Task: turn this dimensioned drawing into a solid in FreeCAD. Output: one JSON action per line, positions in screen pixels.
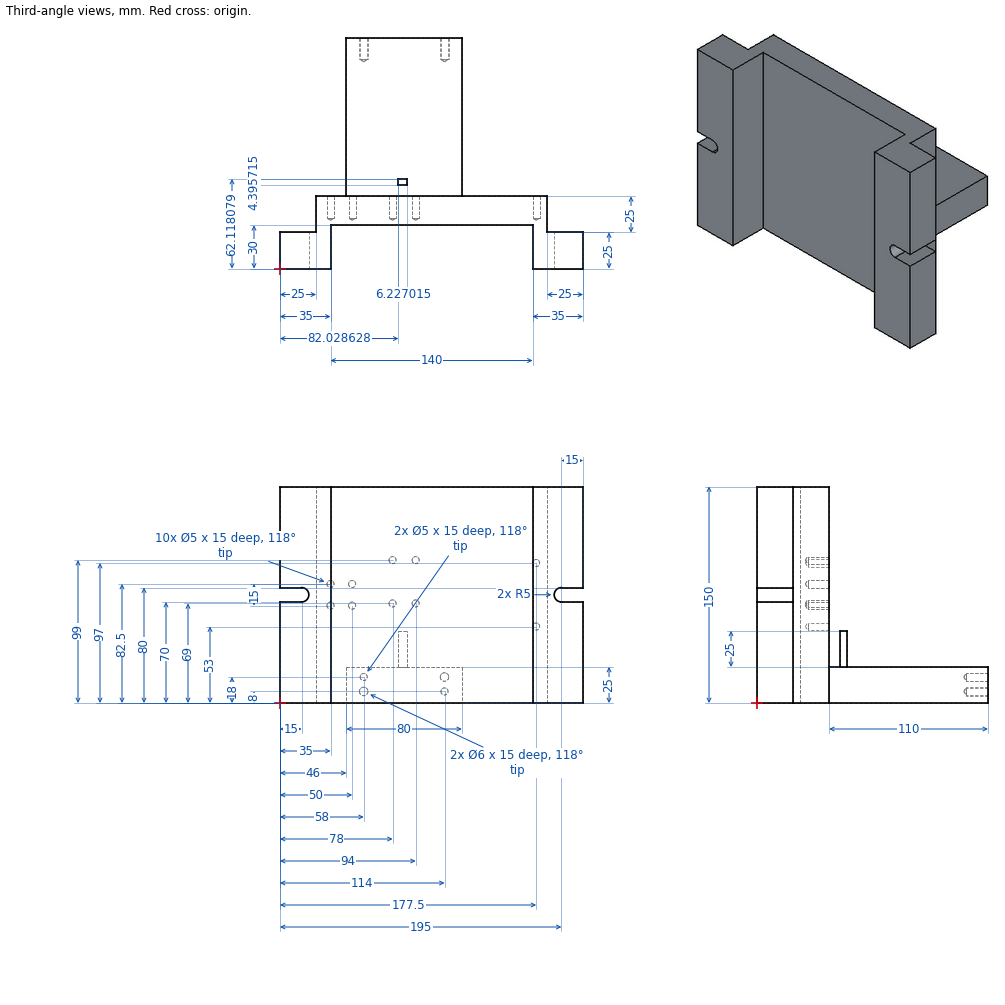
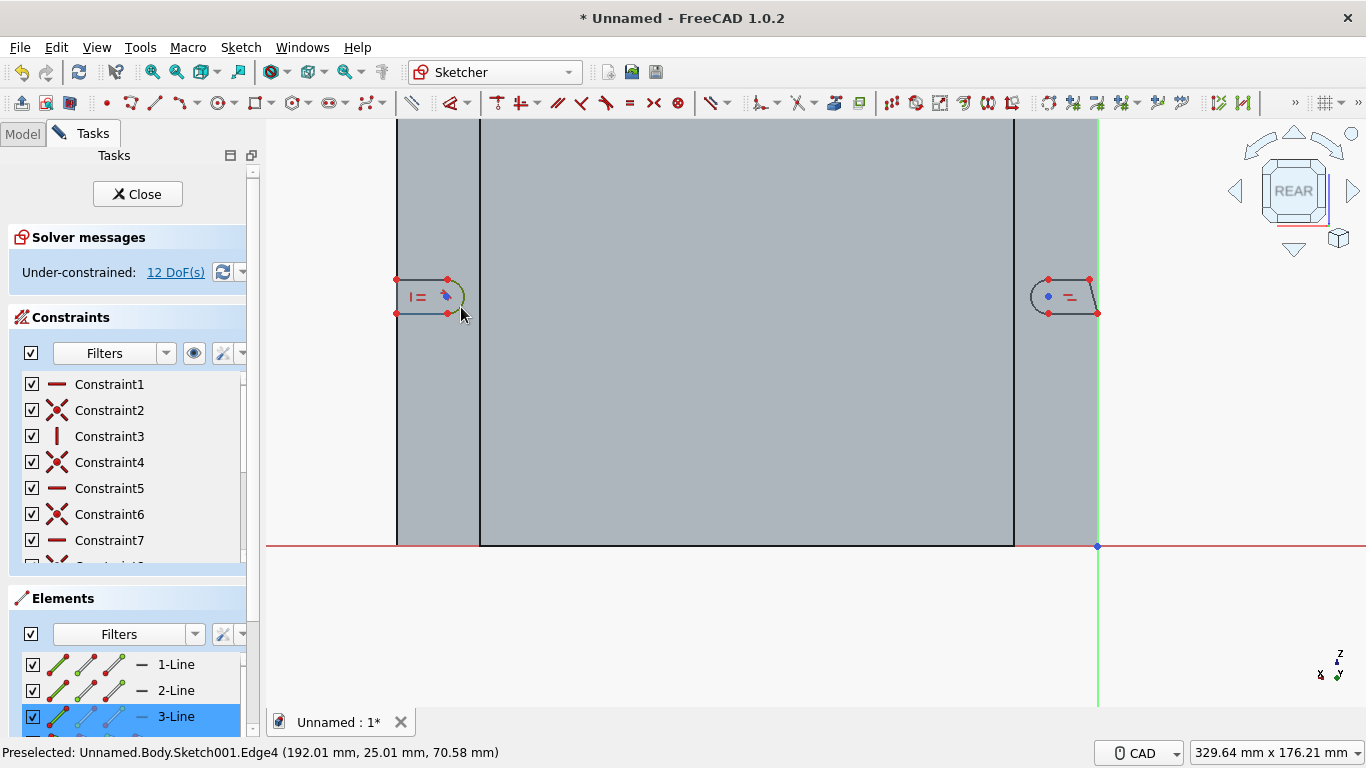
{"action": "key", "text": "t"}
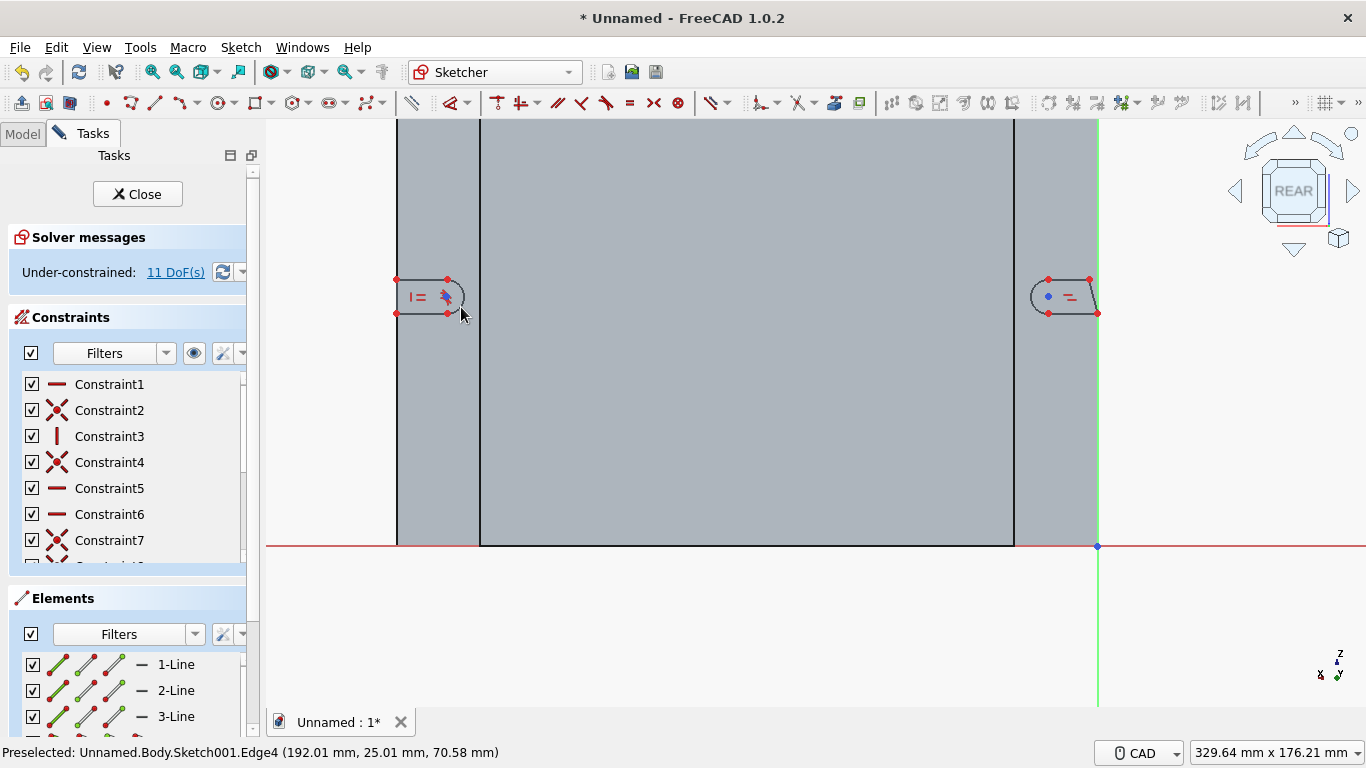
{"action": "left_click", "coordinate": [1063, 314]}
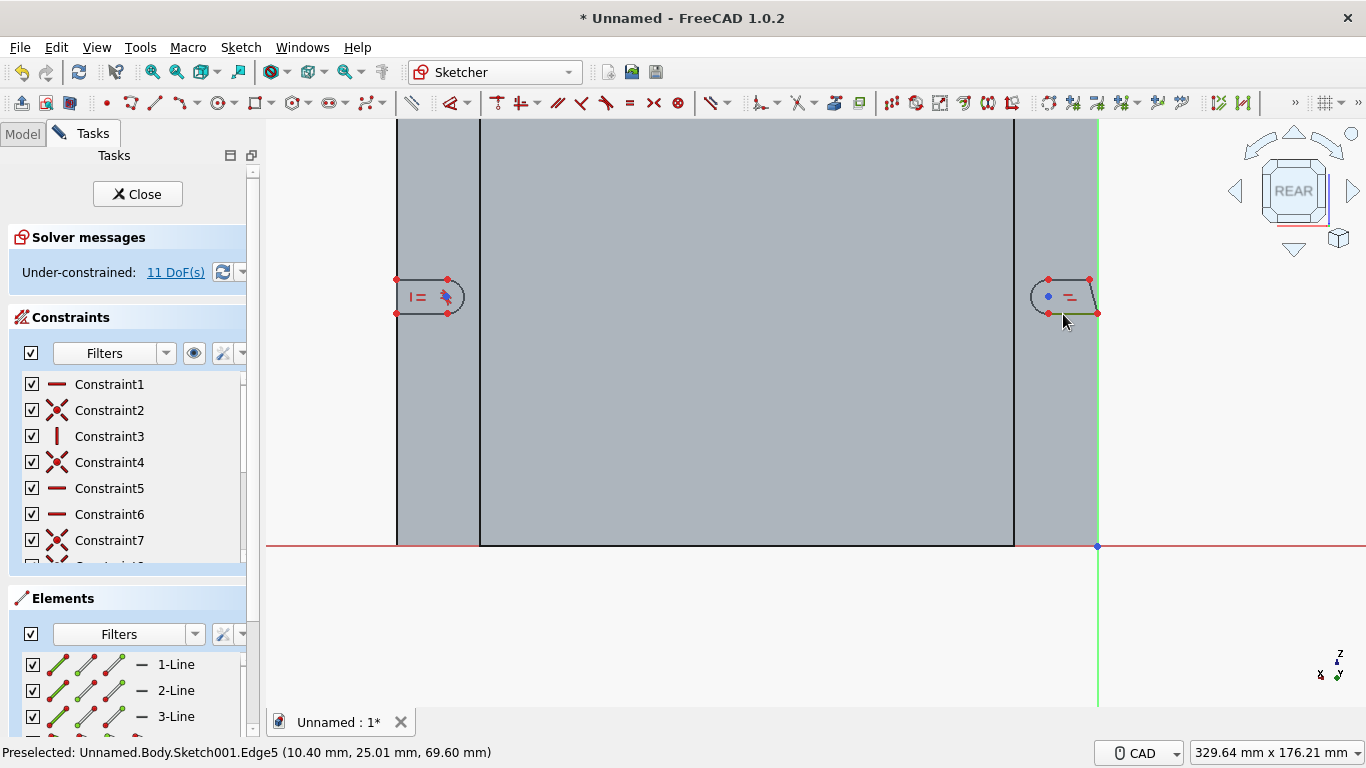
{"action": "left_click", "coordinate": [1034, 287]}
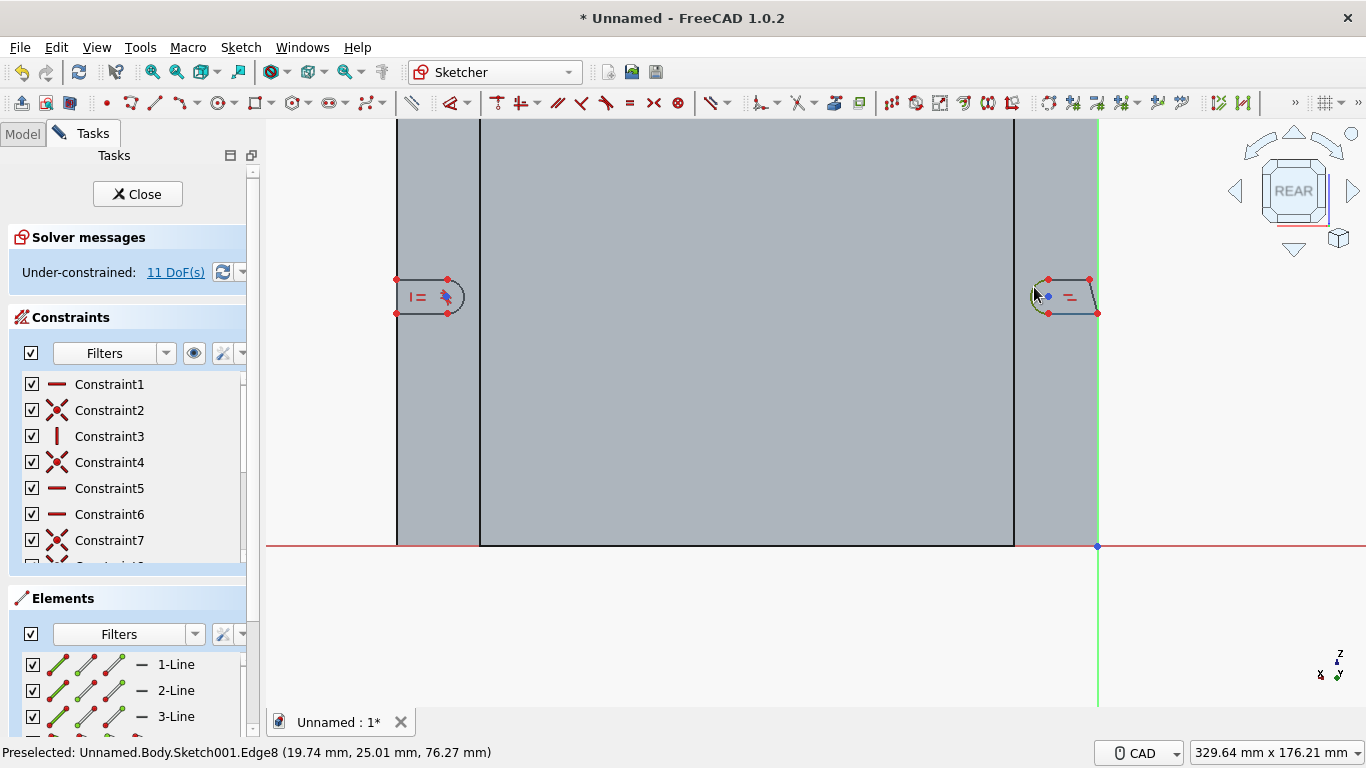
{"action": "left_click", "coordinate": [606, 104]}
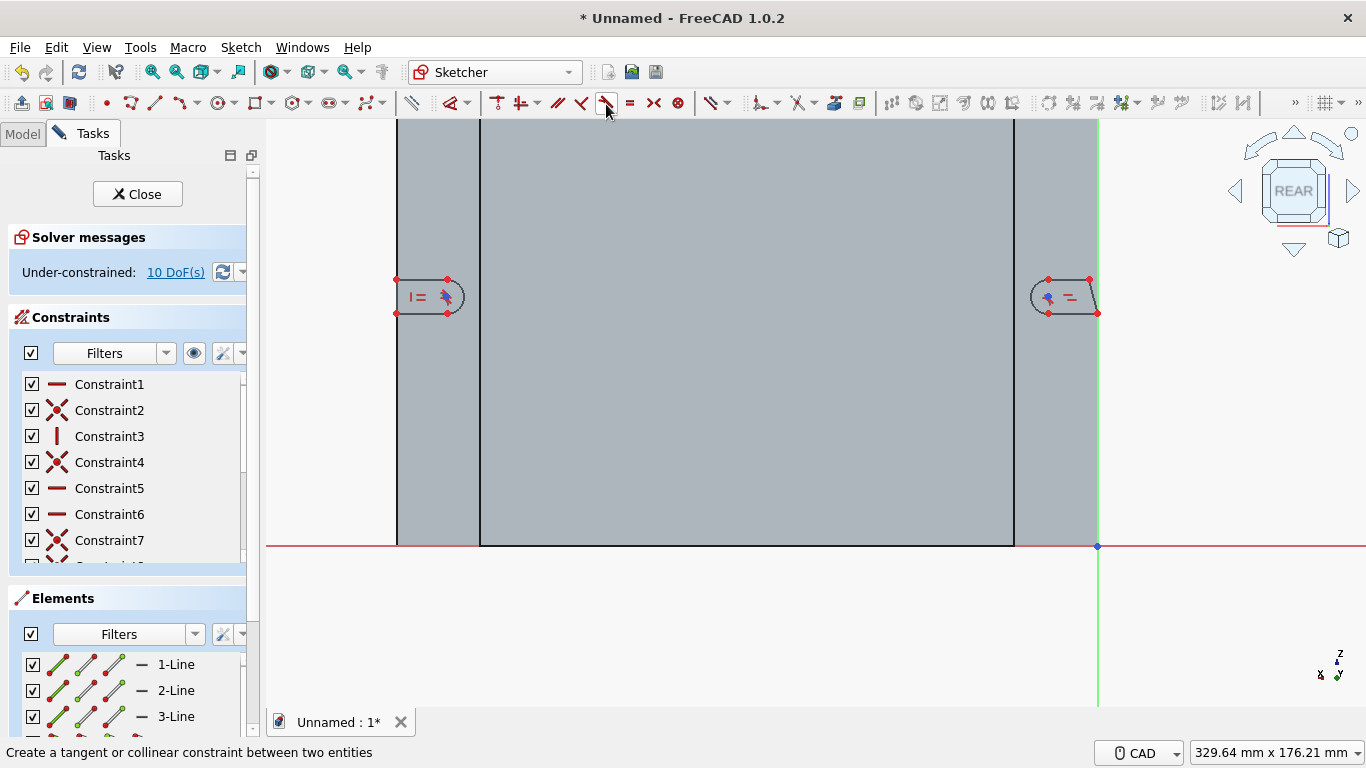
{"action": "left_click", "coordinate": [1077, 280]}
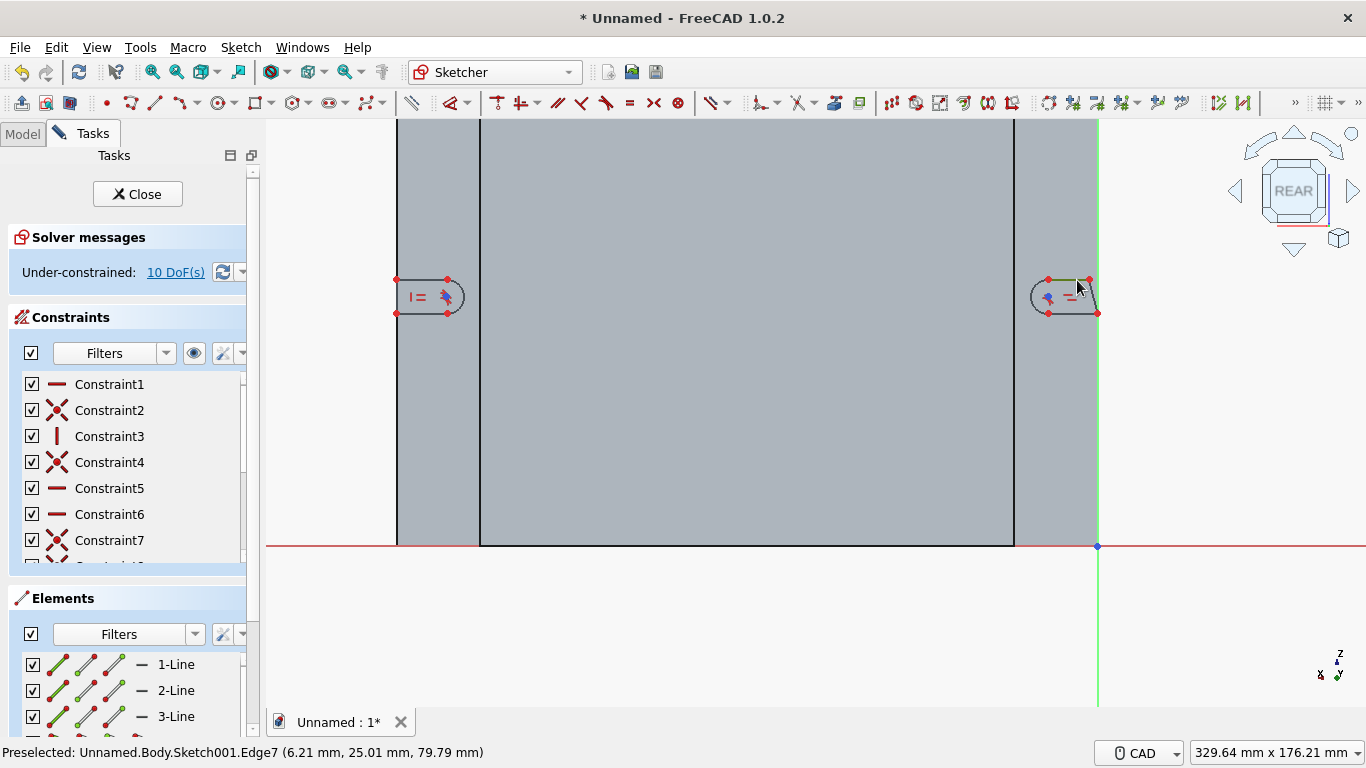
{"action": "left_click", "coordinate": [1034, 287]}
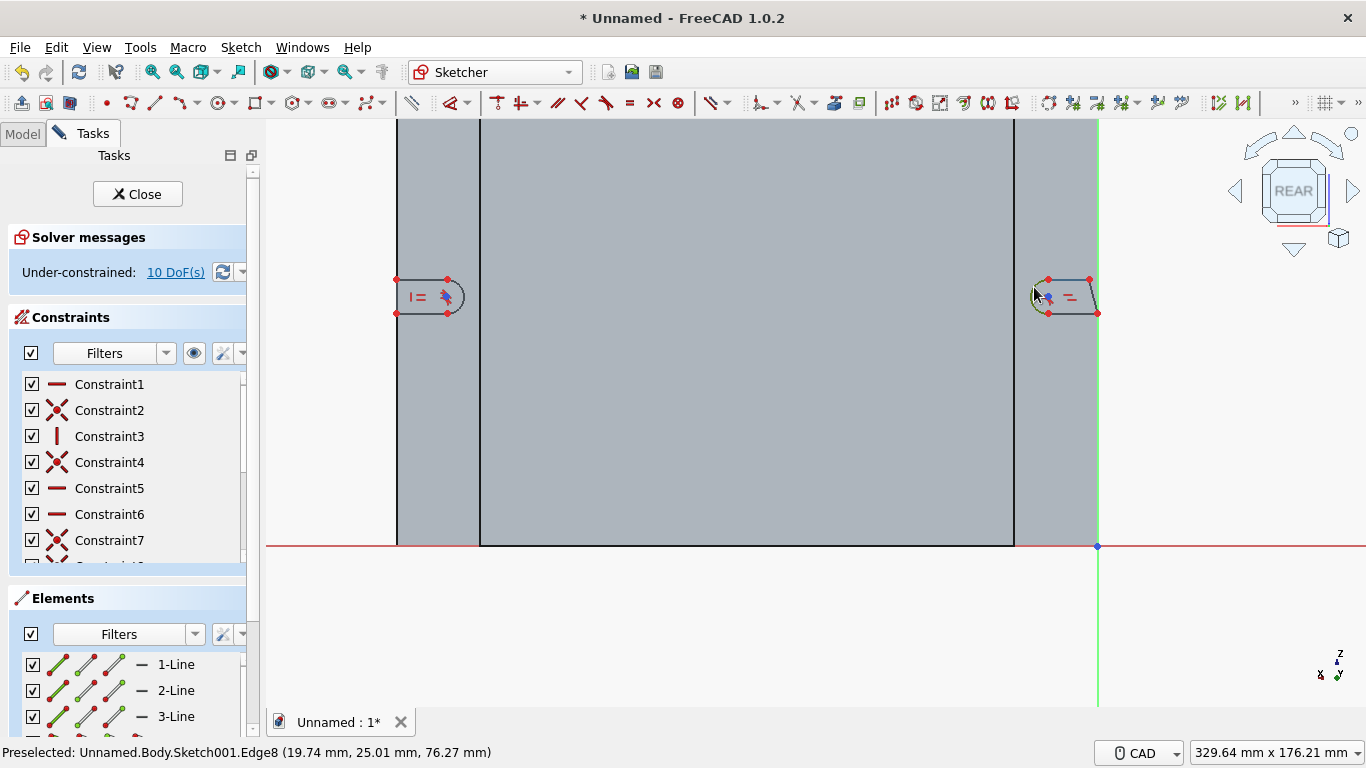
{"action": "key", "text": "t"}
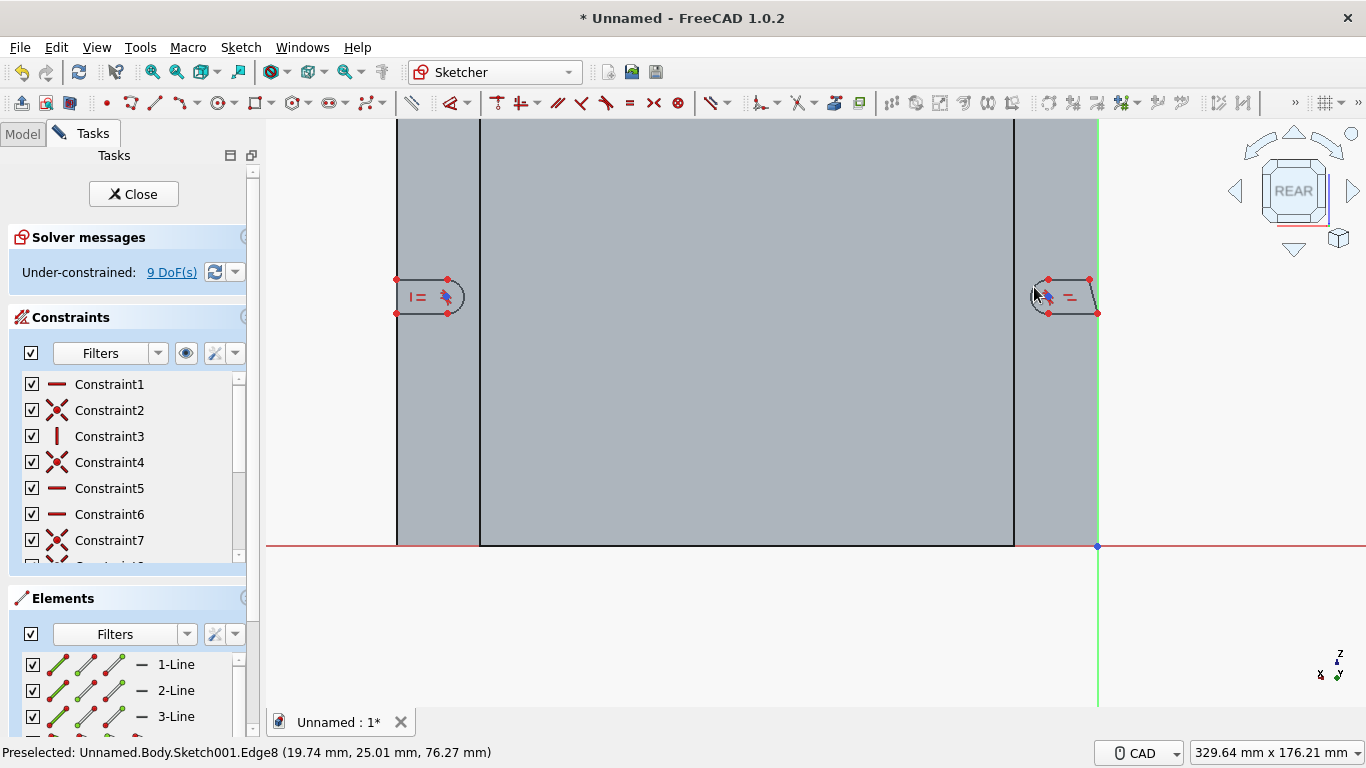
{"action": "scroll", "coordinate": [1095, 304], "scroll_direction": "up", "scroll_amount": 2}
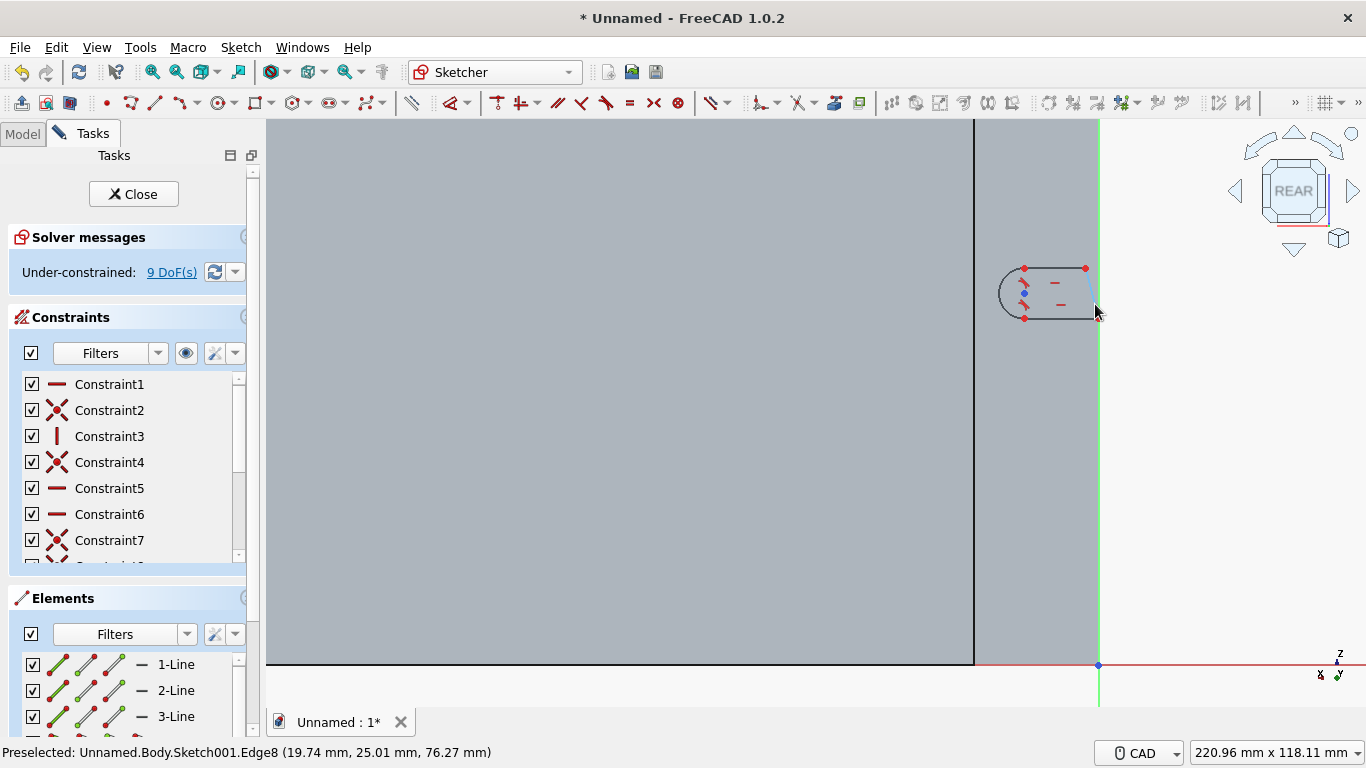
{"action": "left_click", "coordinate": [1095, 304]}